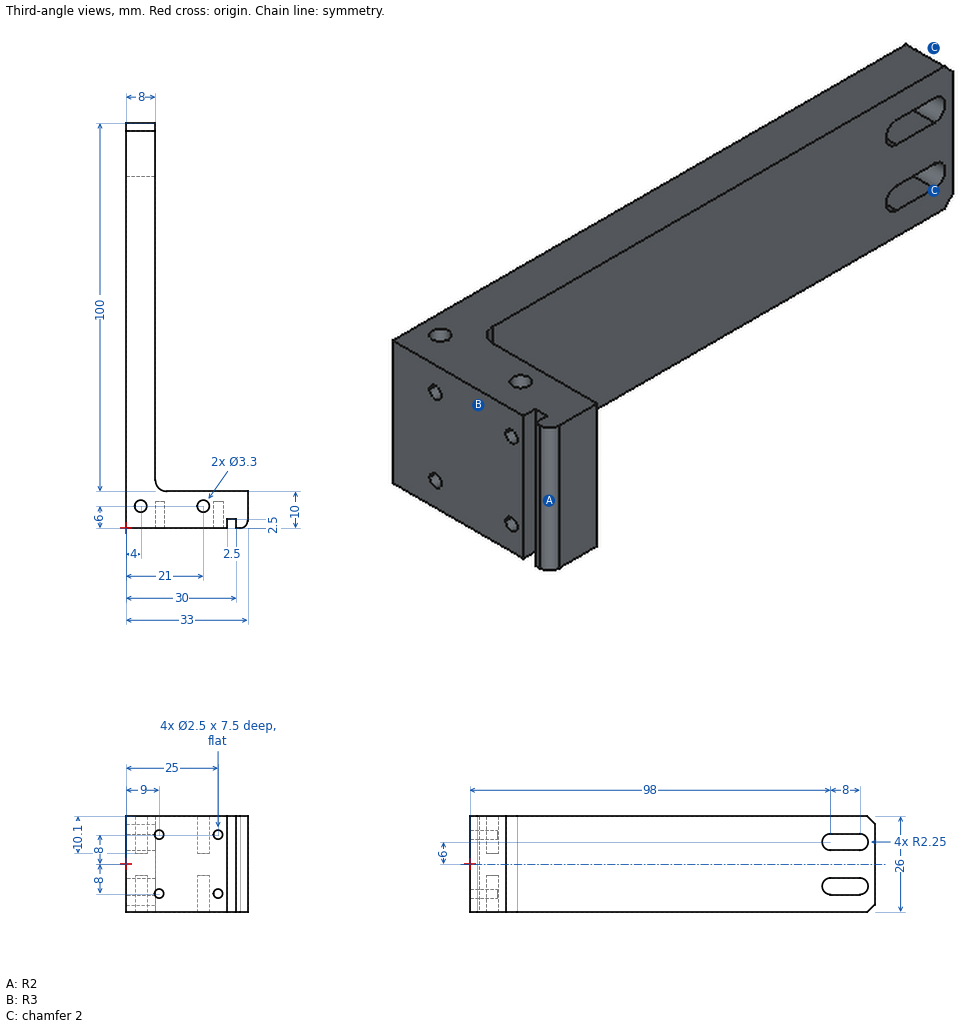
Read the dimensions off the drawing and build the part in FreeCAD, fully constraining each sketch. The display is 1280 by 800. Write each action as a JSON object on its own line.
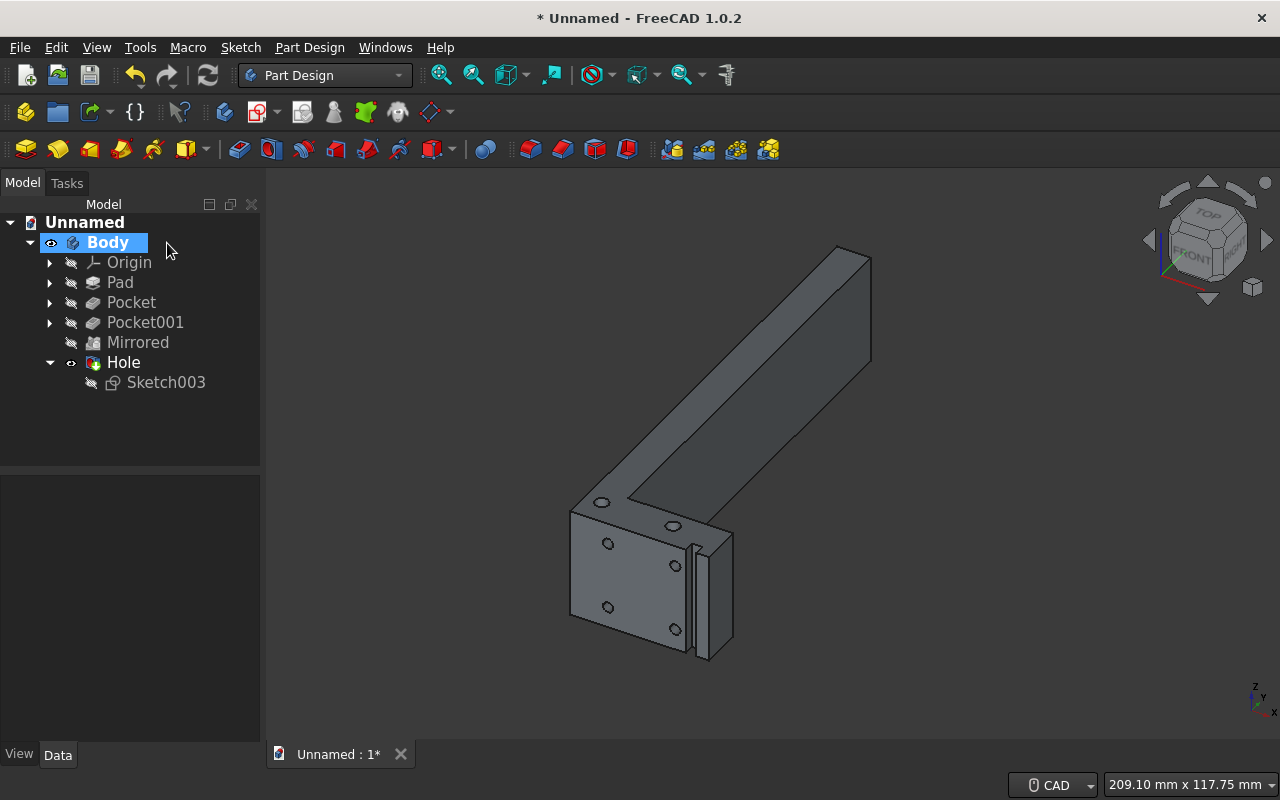
{"action": "left_click", "coordinate": [819, 360]}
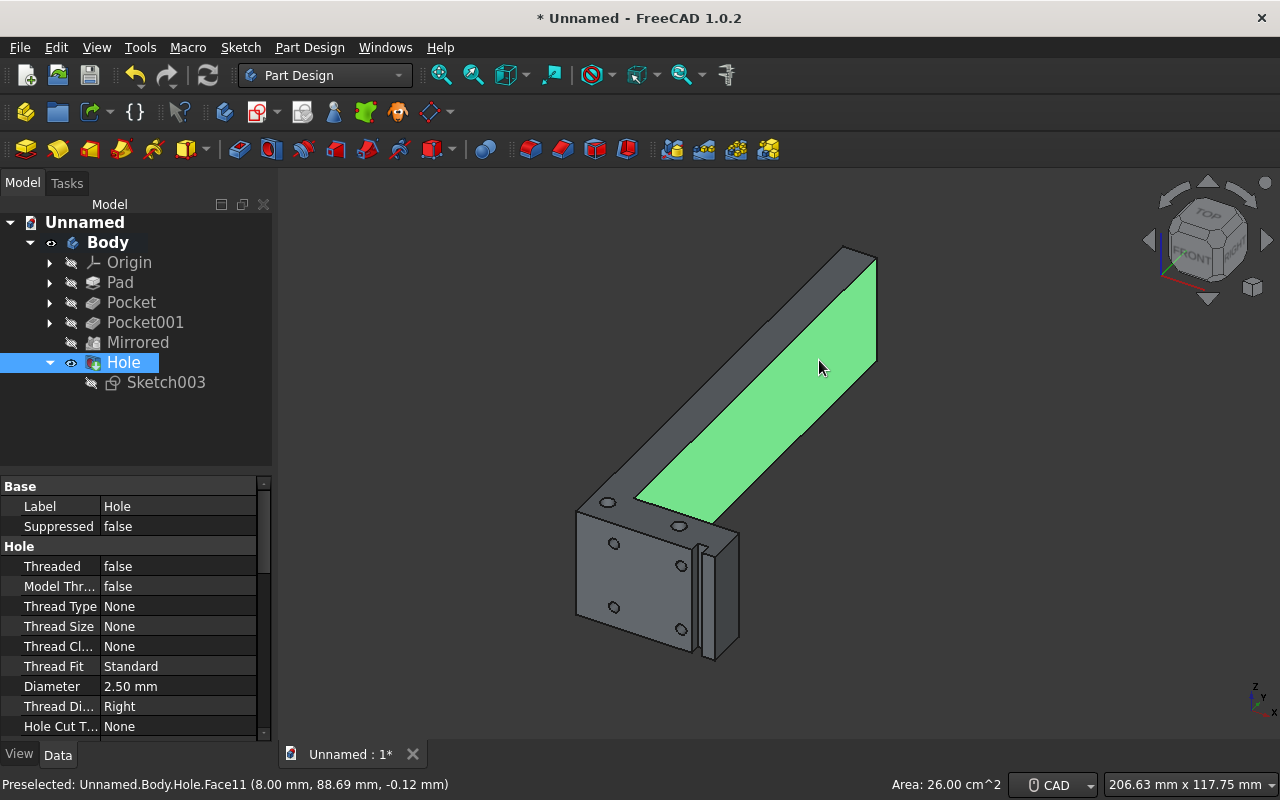
{"action": "left_click", "coordinate": [258, 112]}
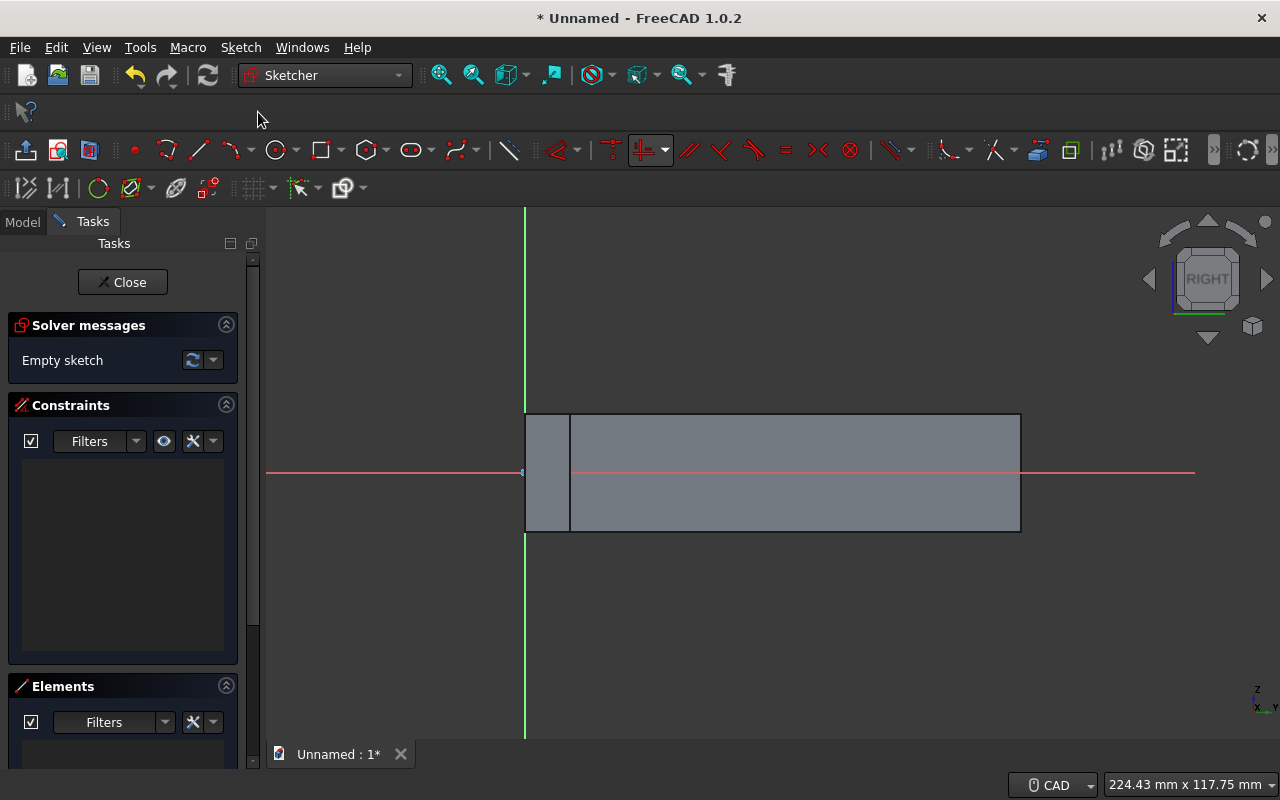
{"action": "left_click", "coordinate": [90, 150]}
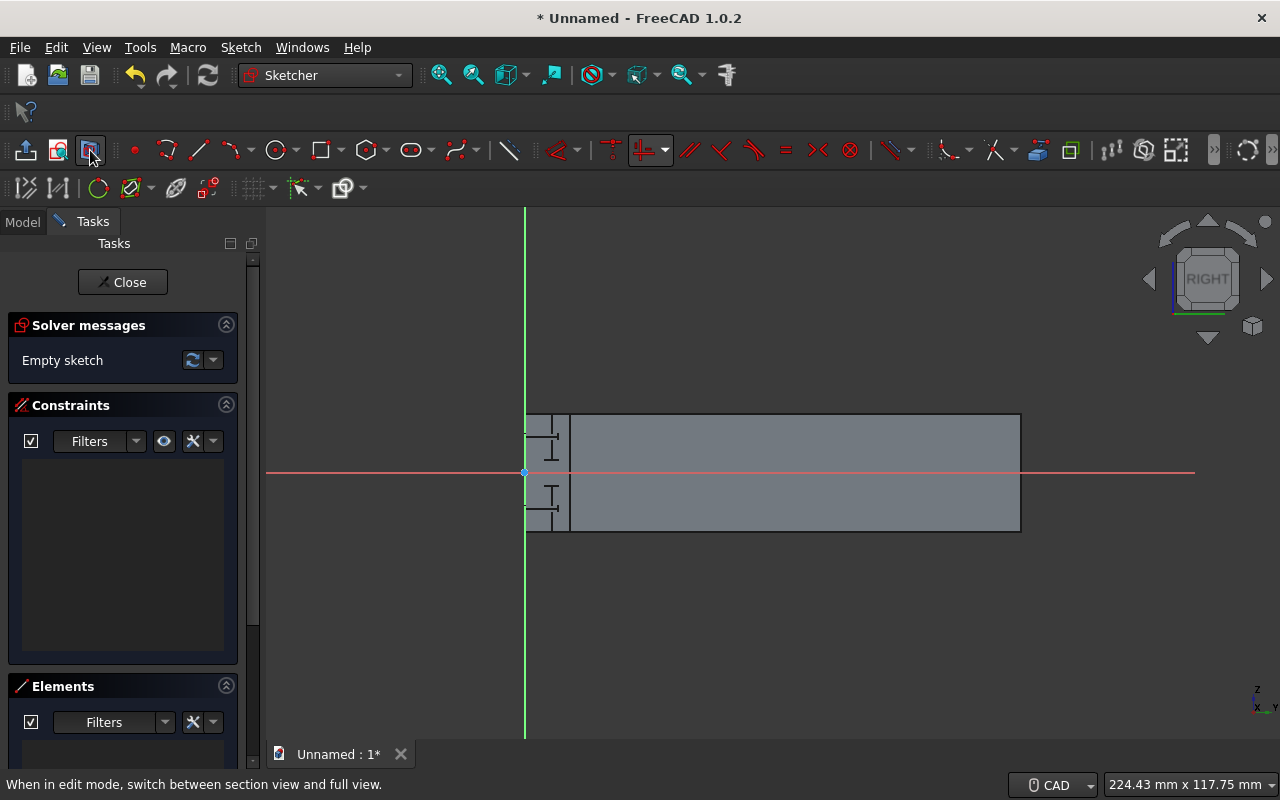
{"action": "scroll", "coordinate": [1056, 473], "scroll_direction": "up", "scroll_amount": 8}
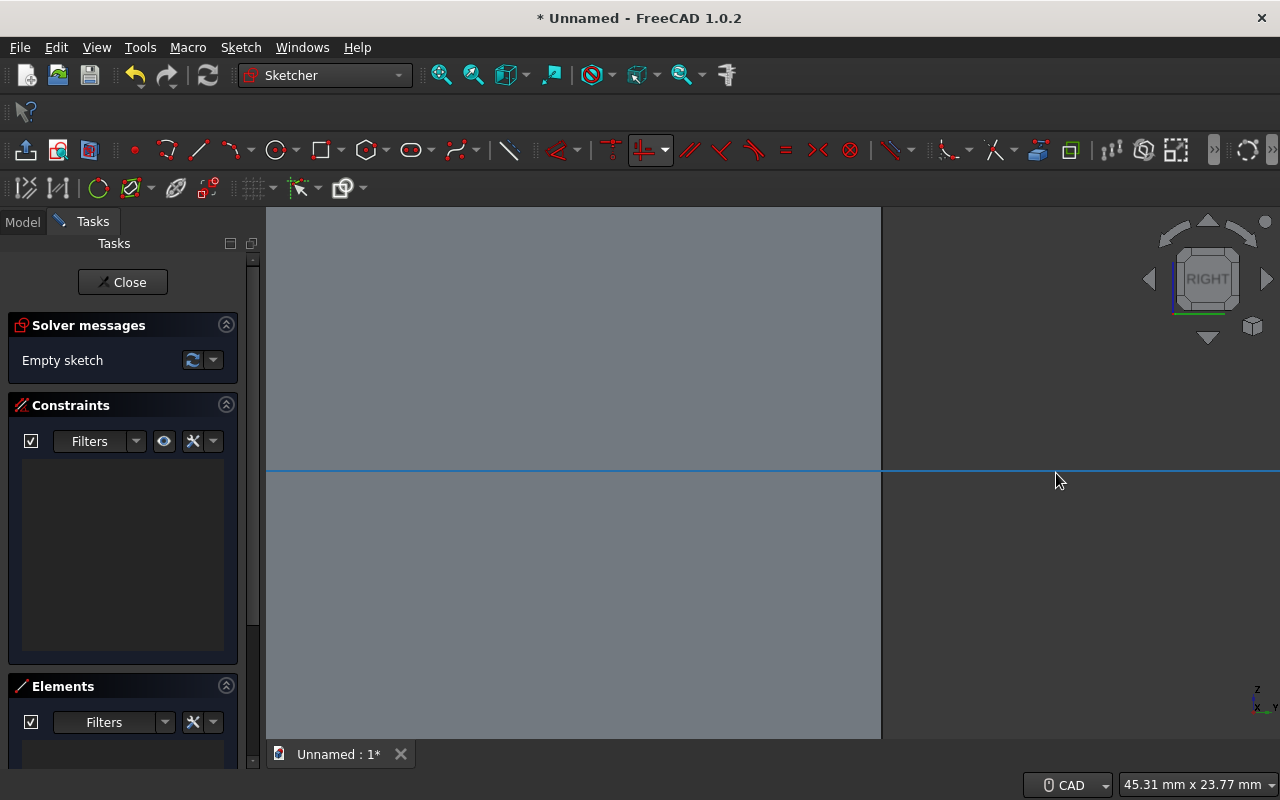
{"action": "left_click", "coordinate": [412, 150]}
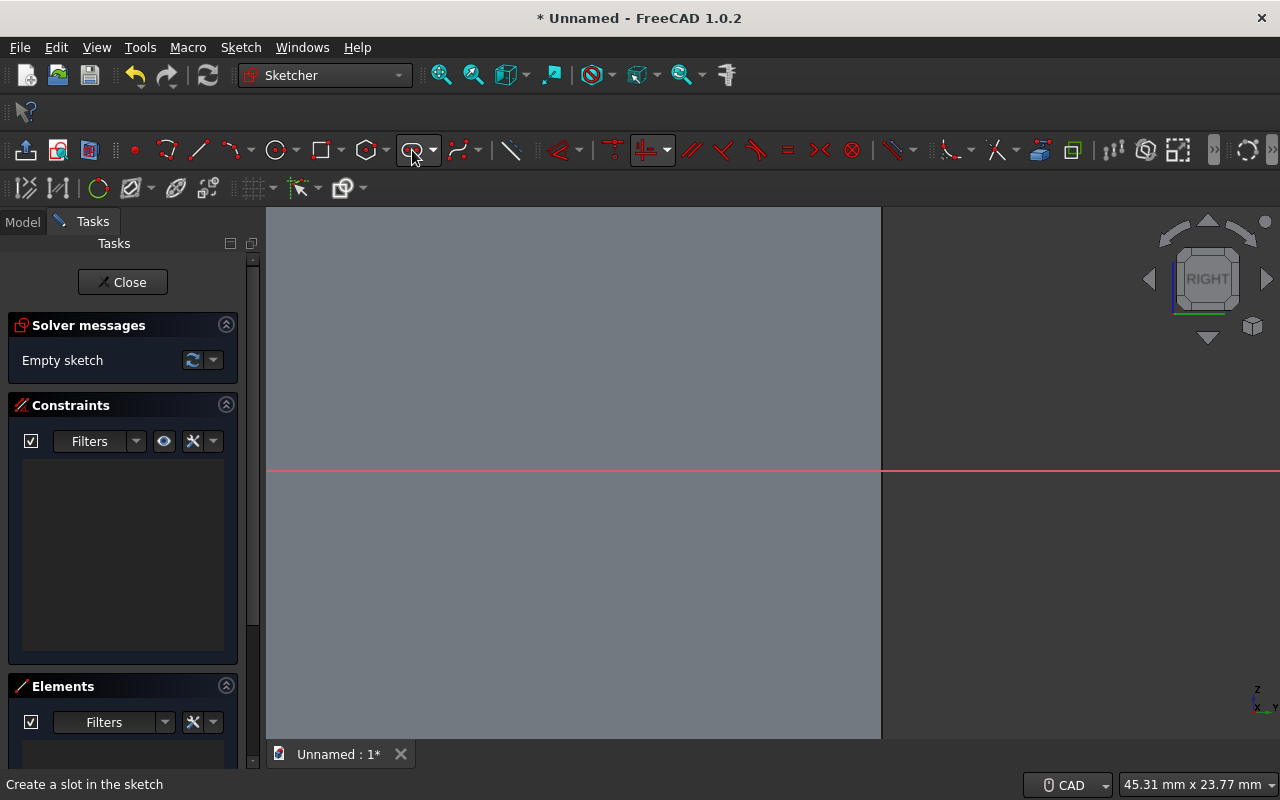
{"action": "left_click", "coordinate": [613, 337]}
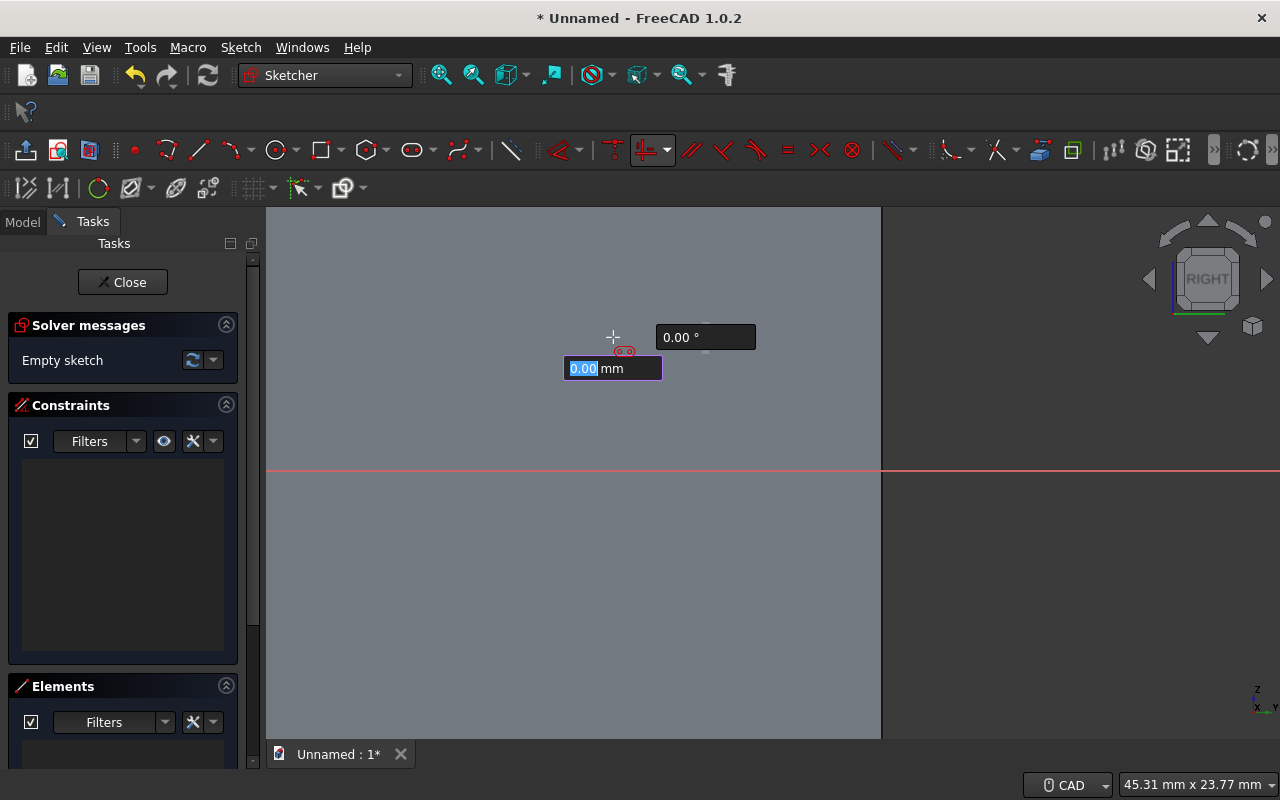
{"action": "left_click", "coordinate": [792, 337]}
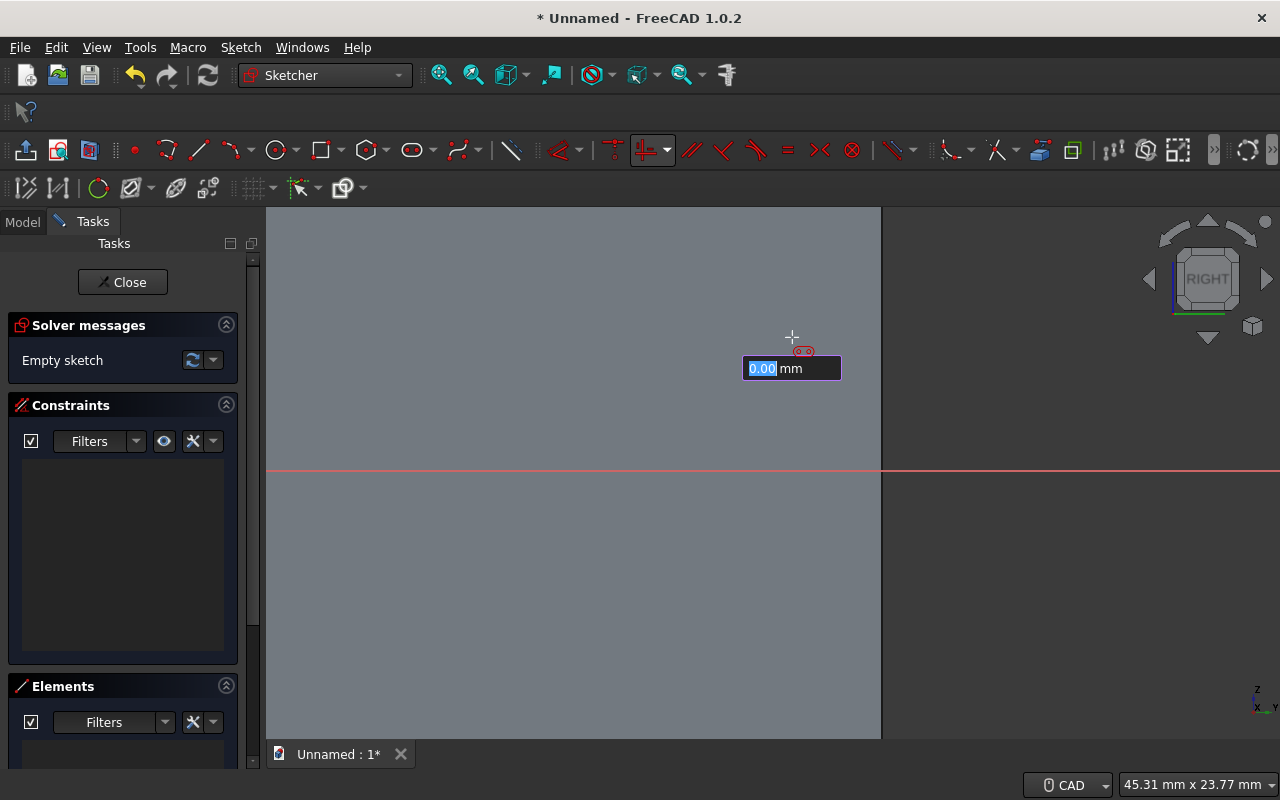
{"action": "left_click", "coordinate": [703, 387]}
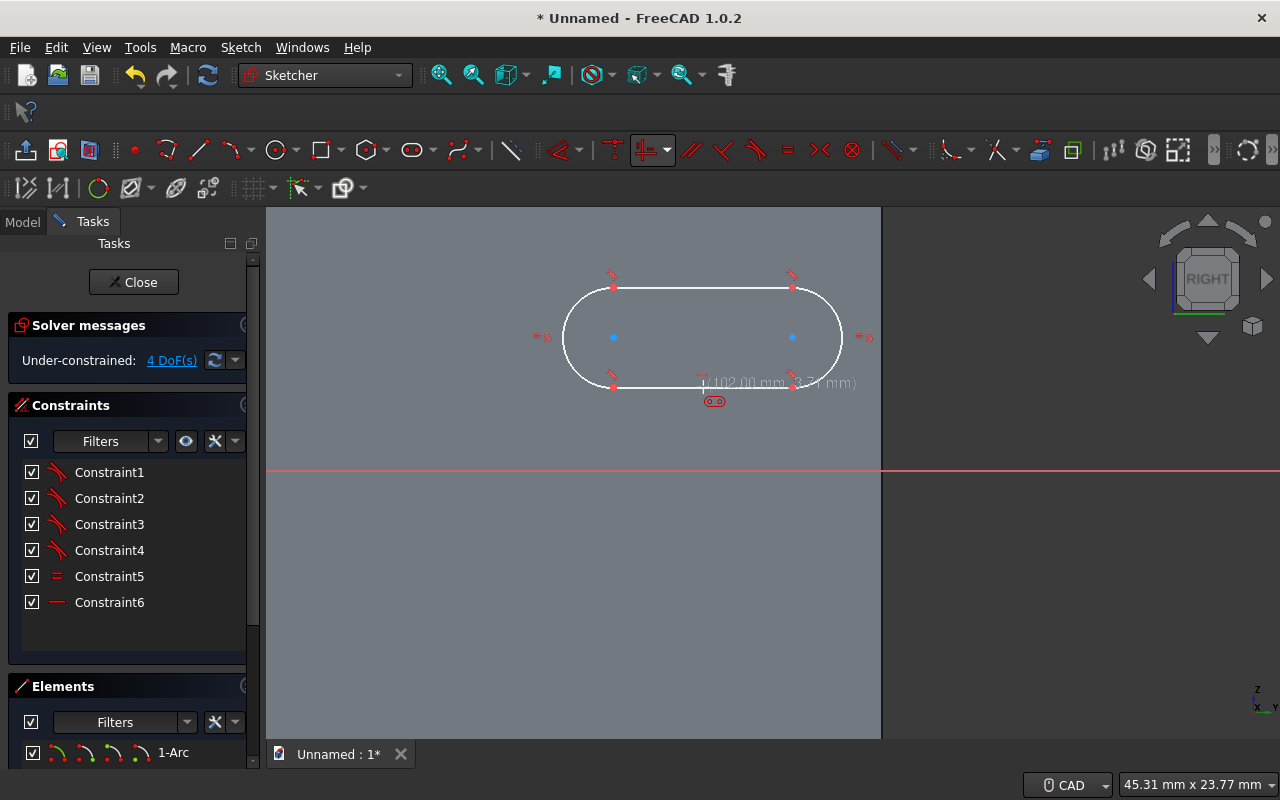
{"action": "left_click", "coordinate": [613, 605]}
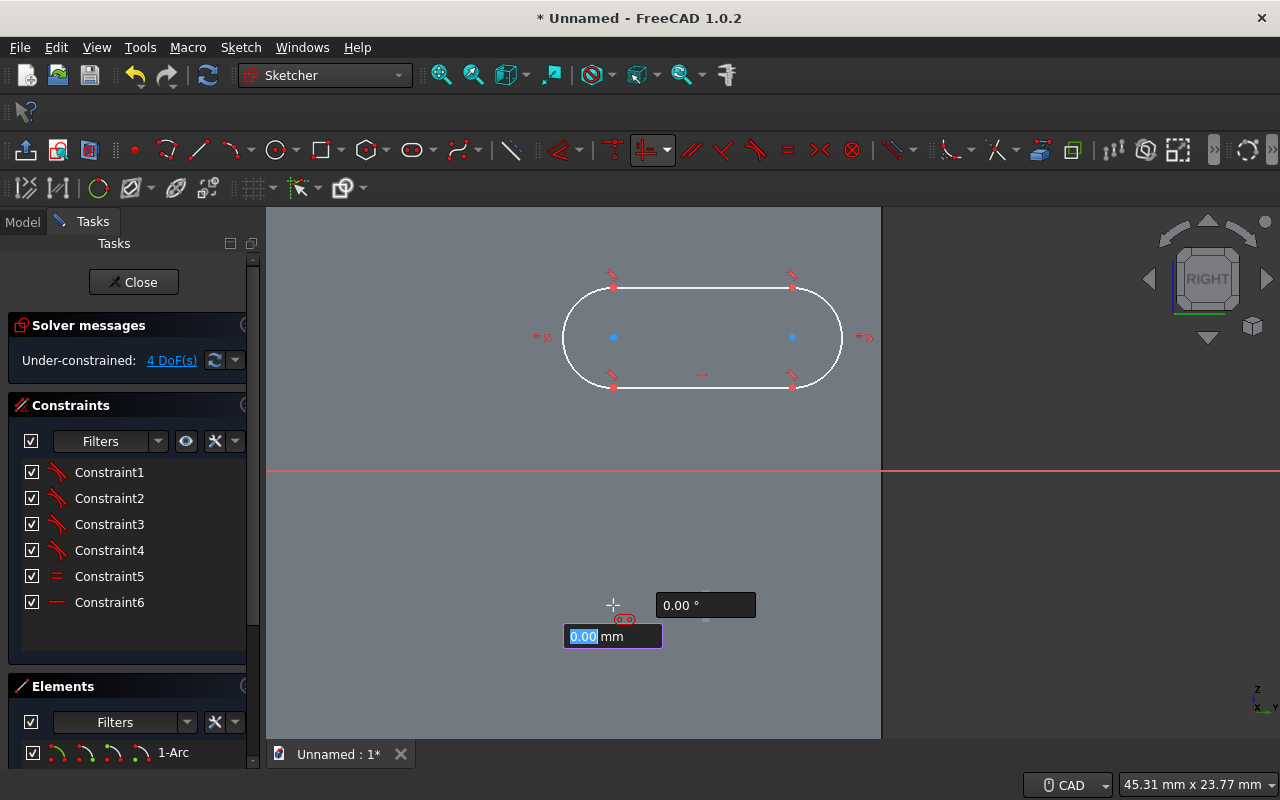
{"action": "left_click", "coordinate": [792, 605]}